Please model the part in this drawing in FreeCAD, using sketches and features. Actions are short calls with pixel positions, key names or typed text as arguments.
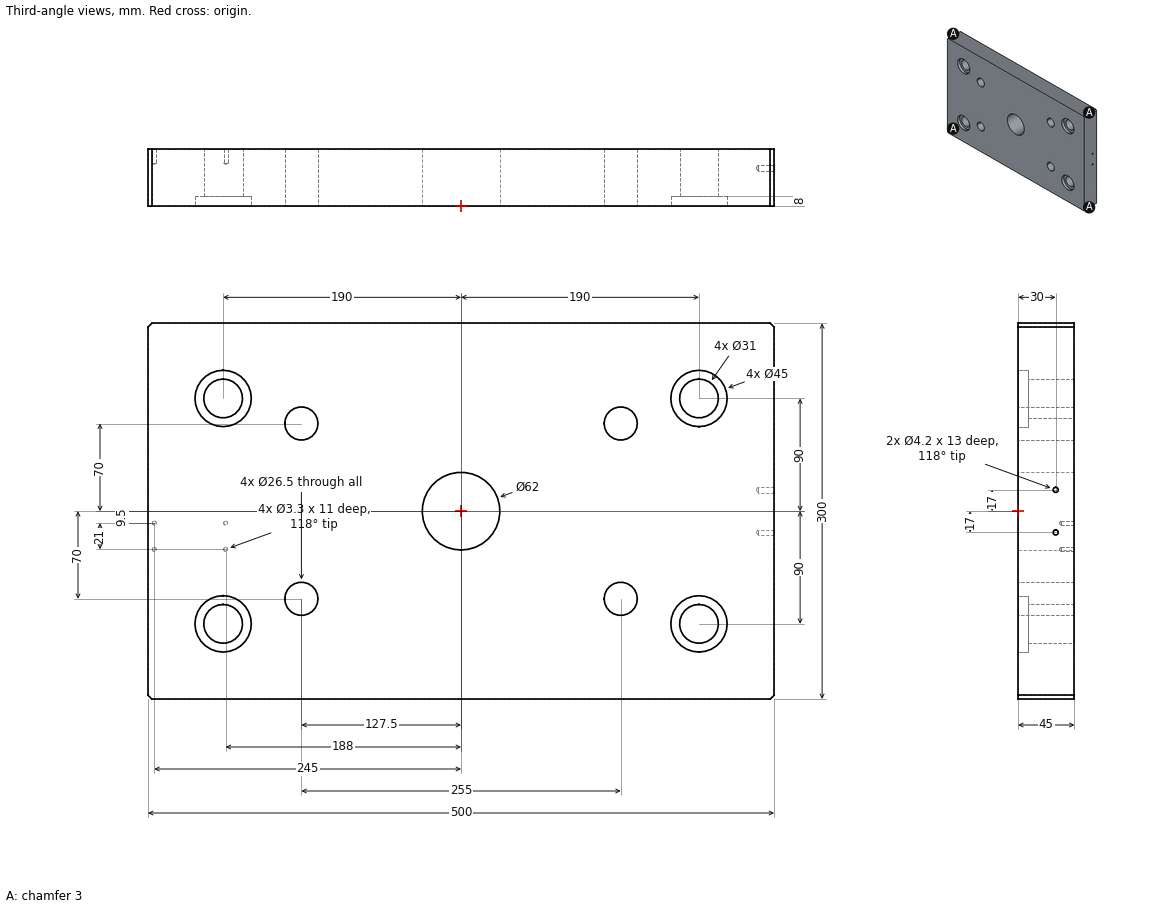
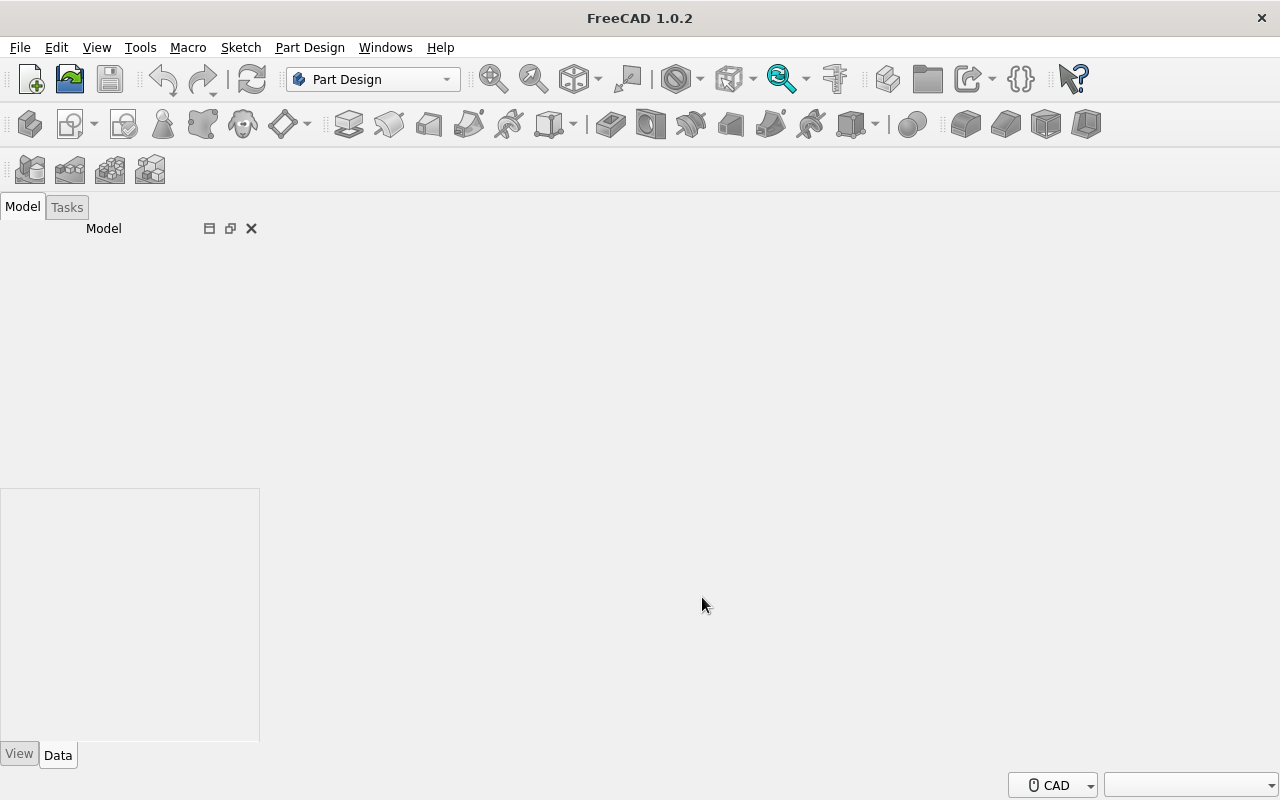
click(30, 80)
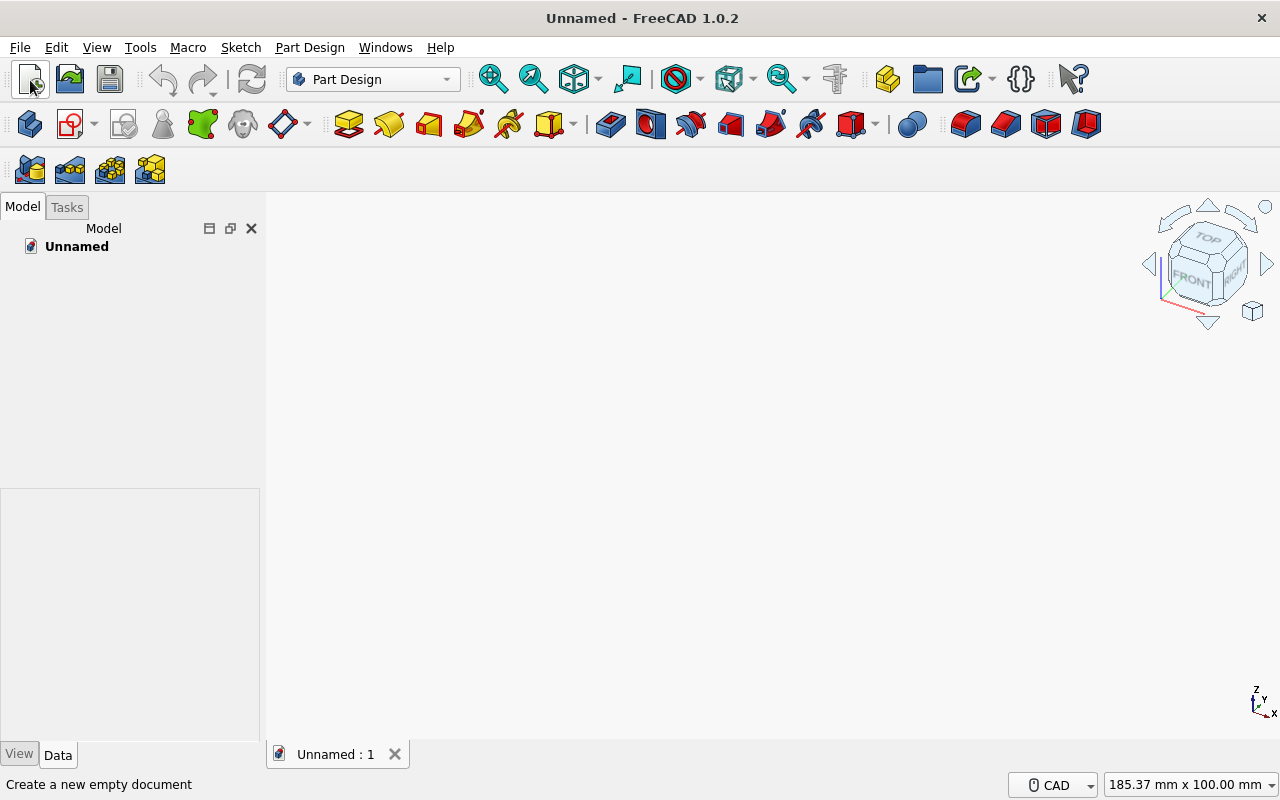
click(70, 124)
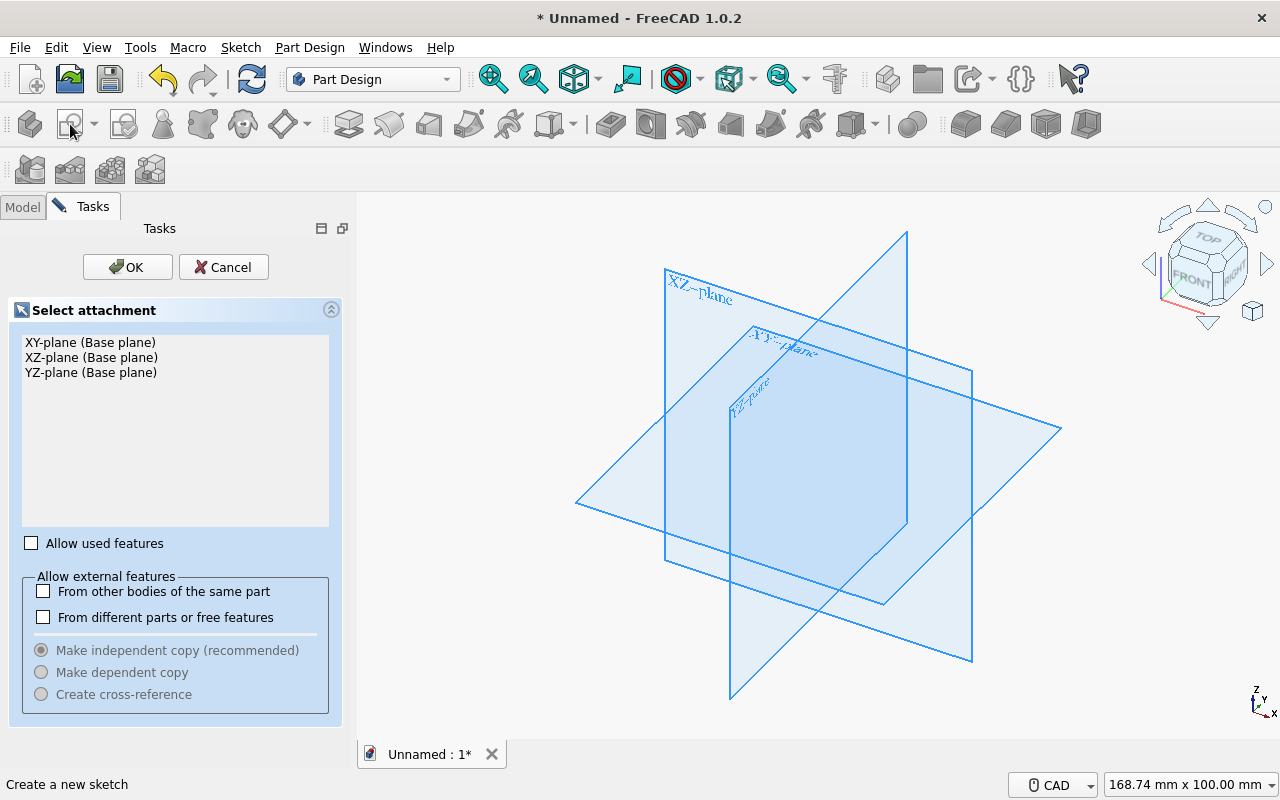
click(82, 358)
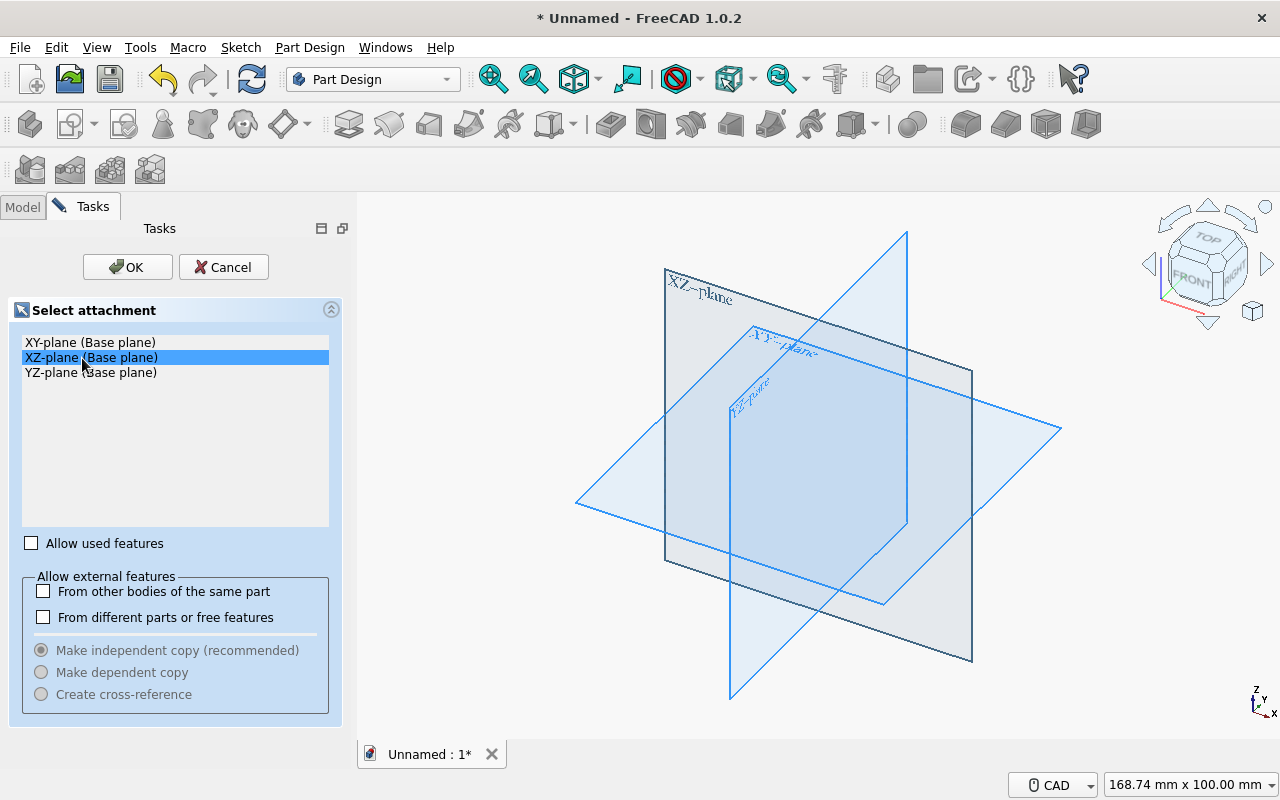
click(128, 267)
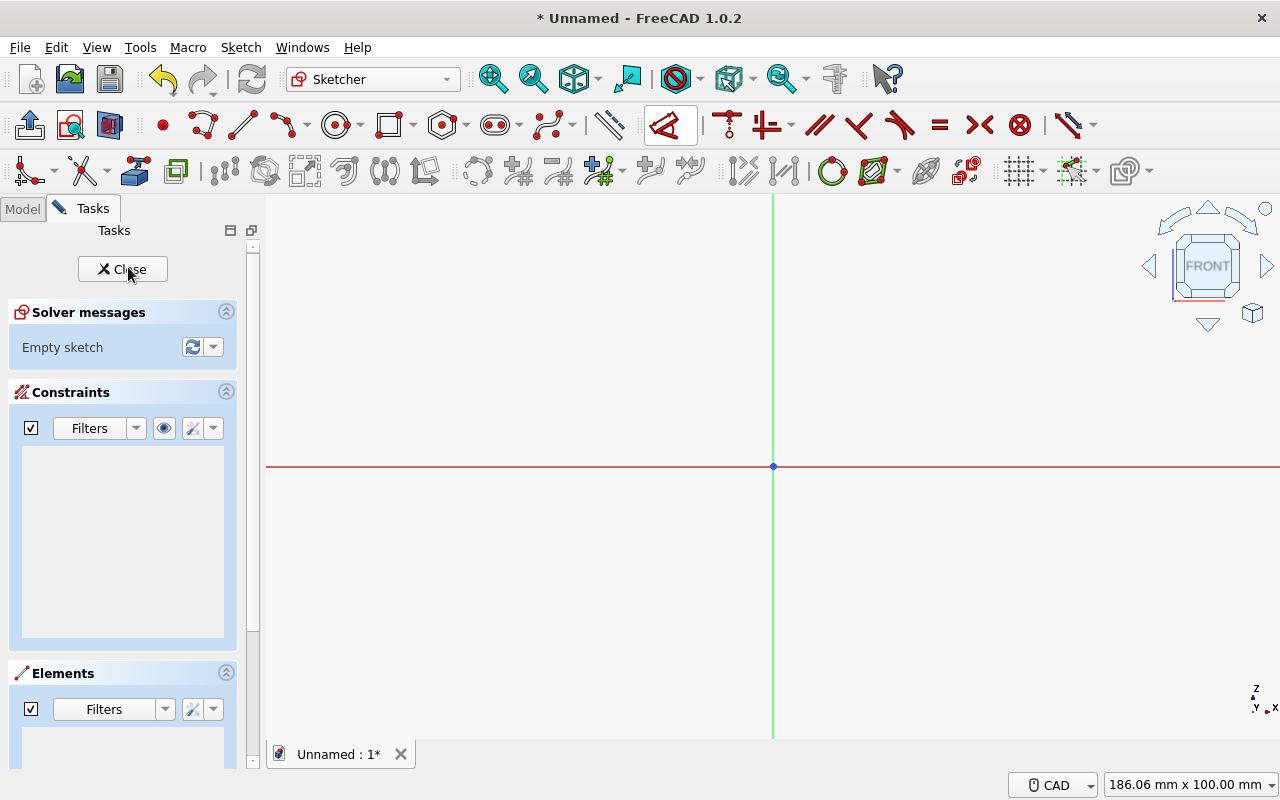
scroll(687, 466, down, 8)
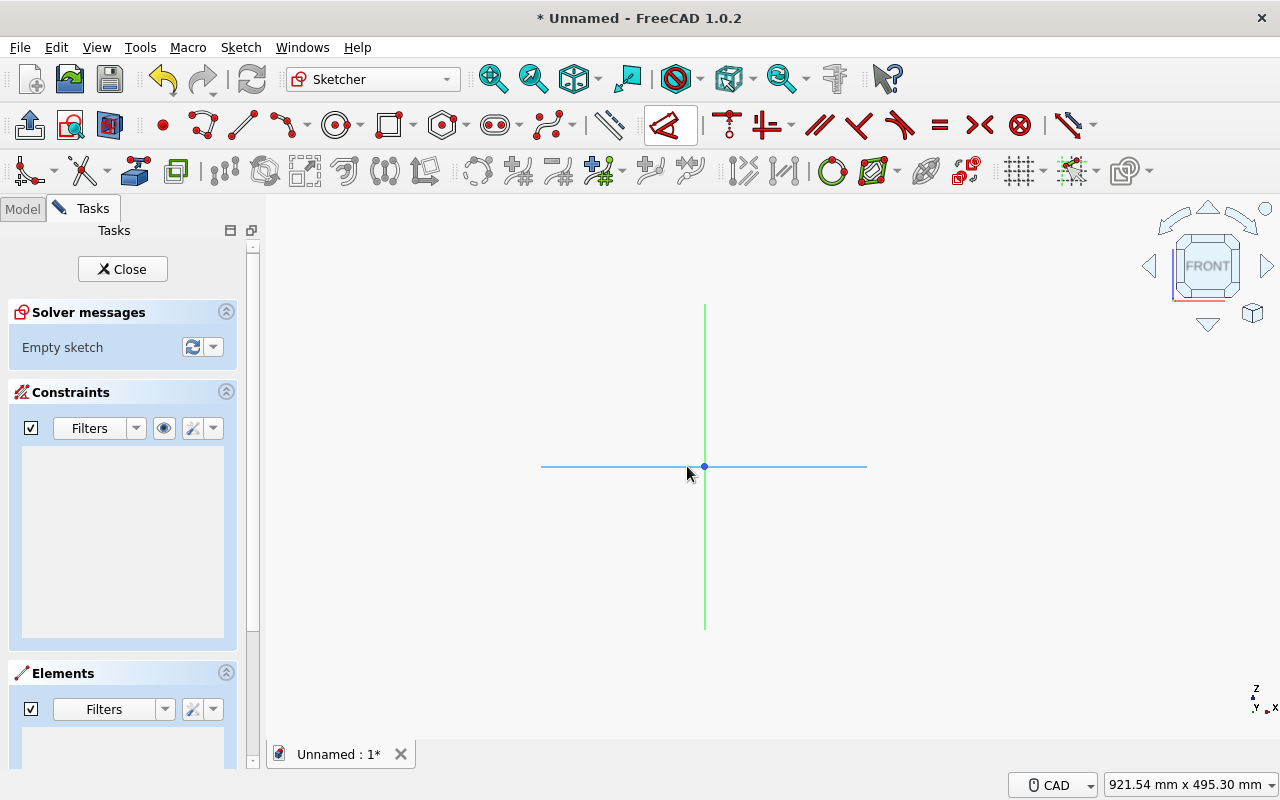
click(416, 126)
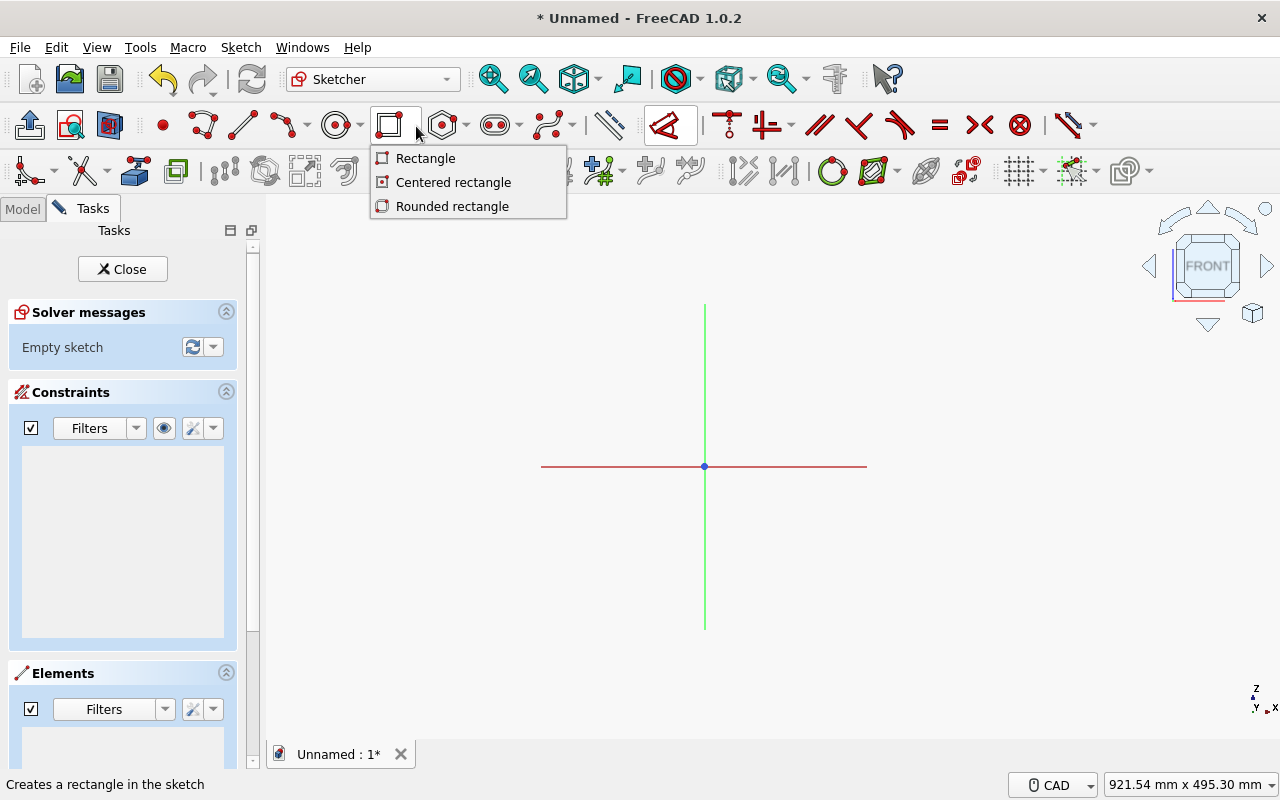
click(468, 182)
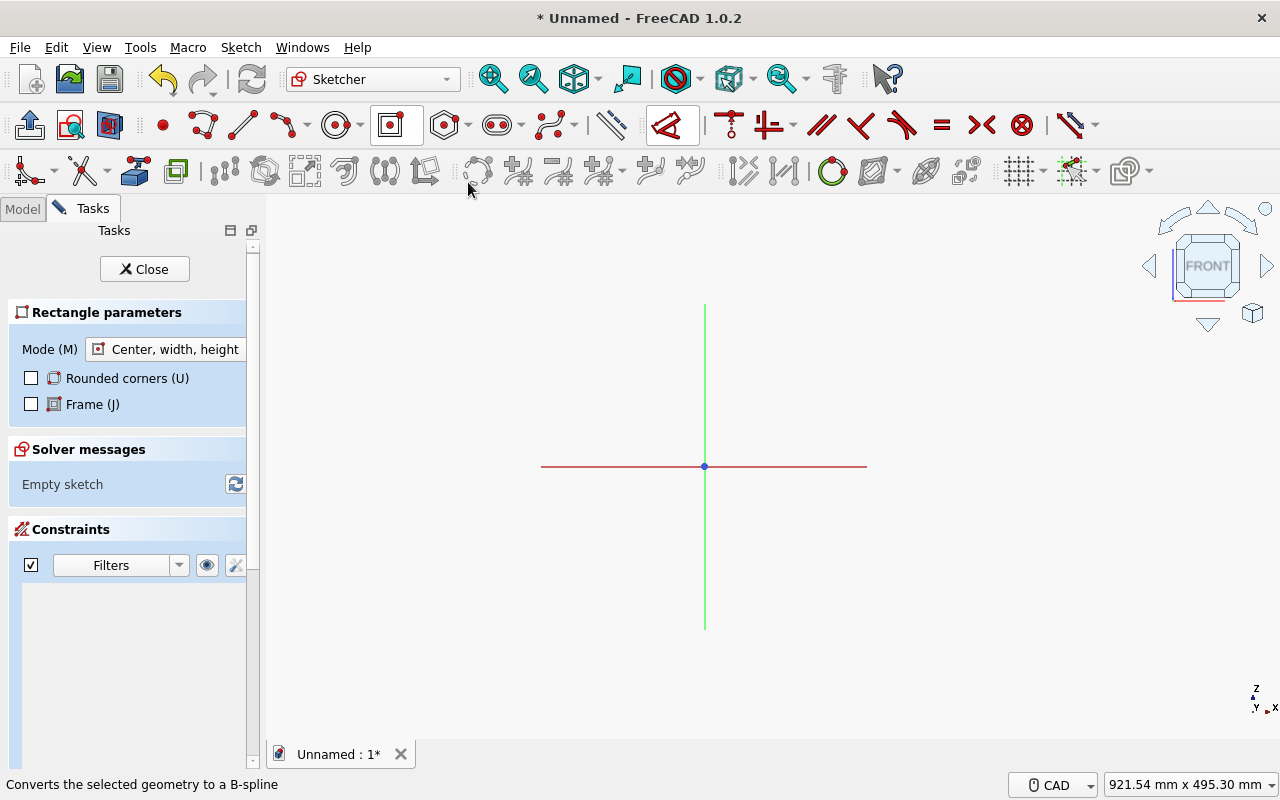
click(705, 466)
click(980, 301)
key(Escape)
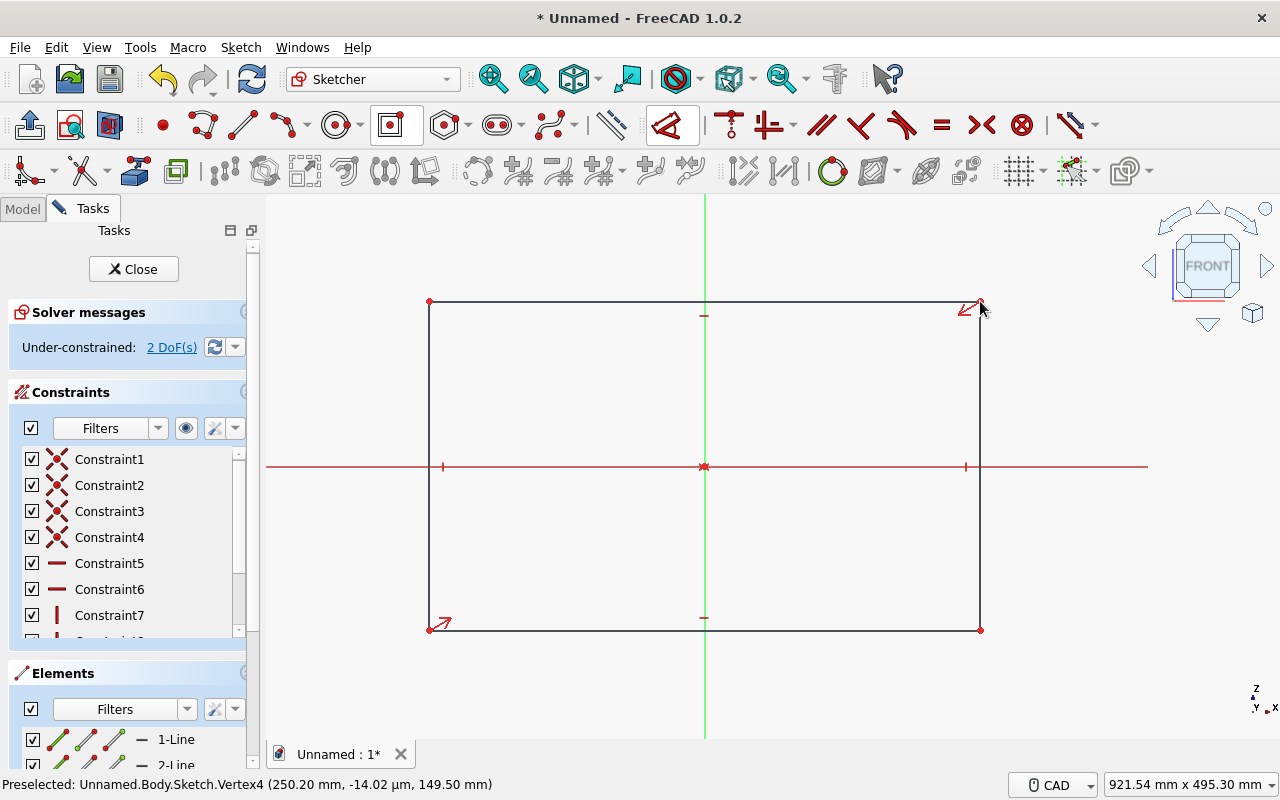
click(666, 126)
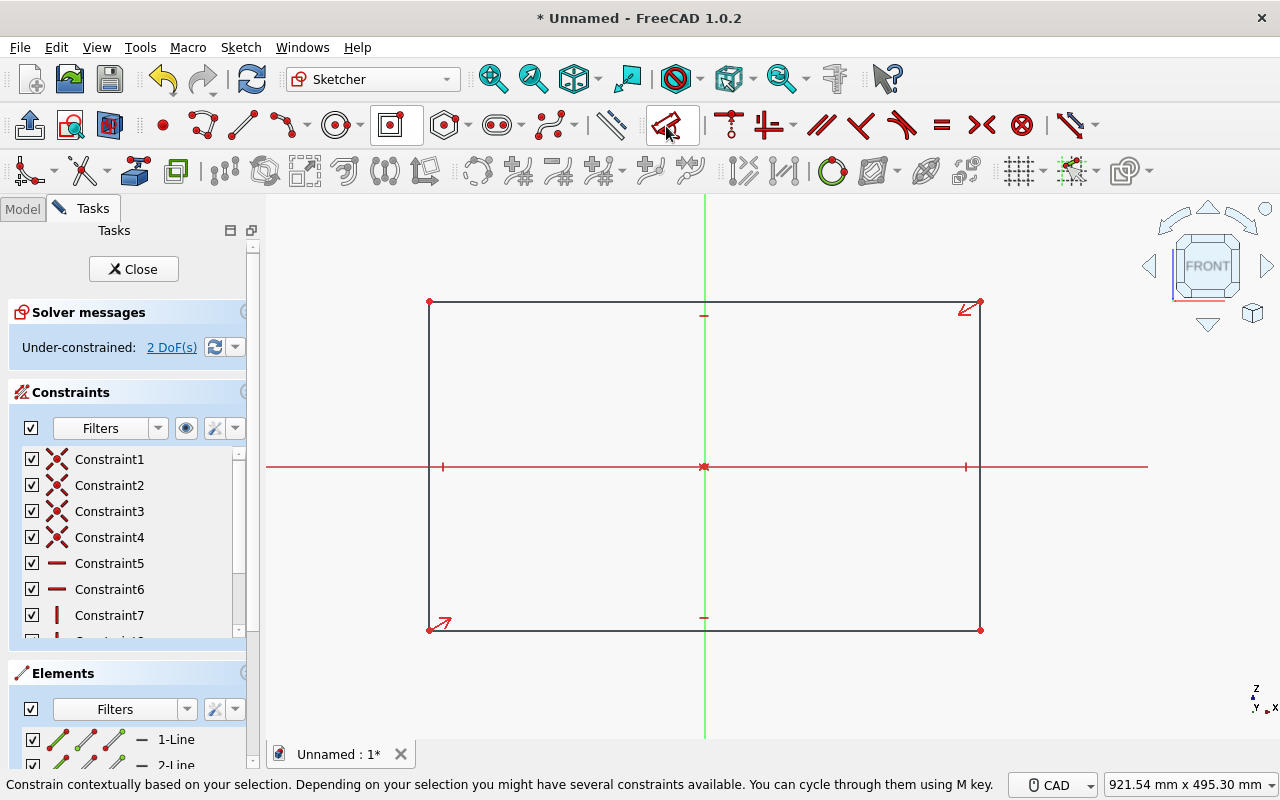
click(595, 631)
click(578, 665)